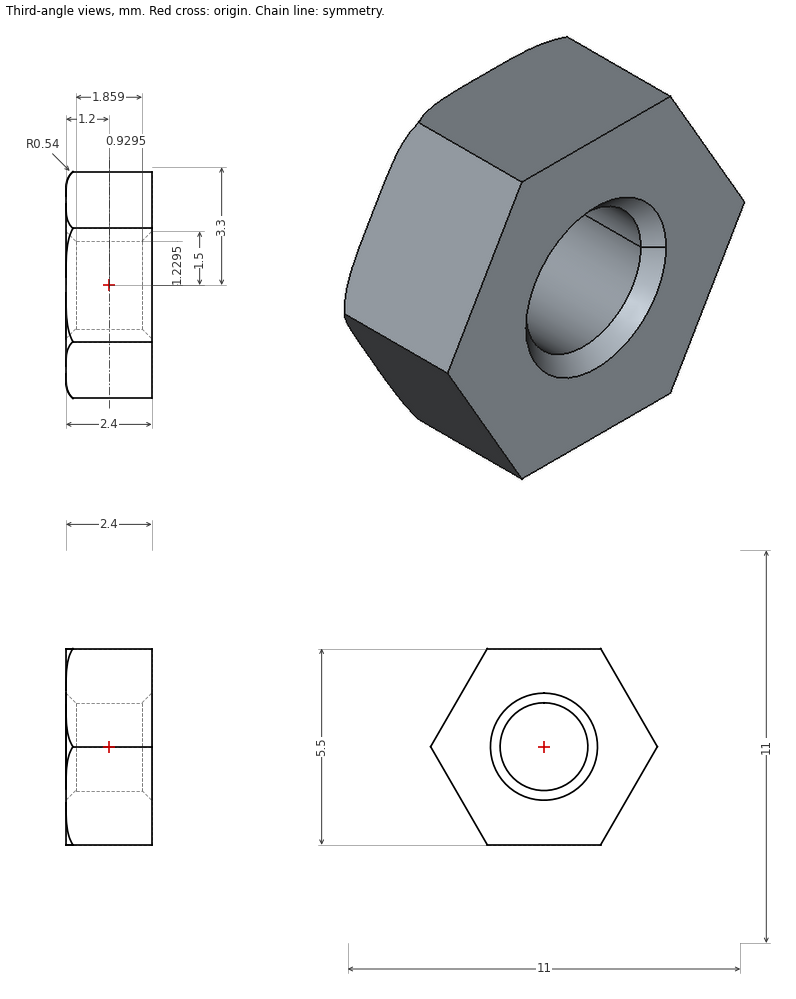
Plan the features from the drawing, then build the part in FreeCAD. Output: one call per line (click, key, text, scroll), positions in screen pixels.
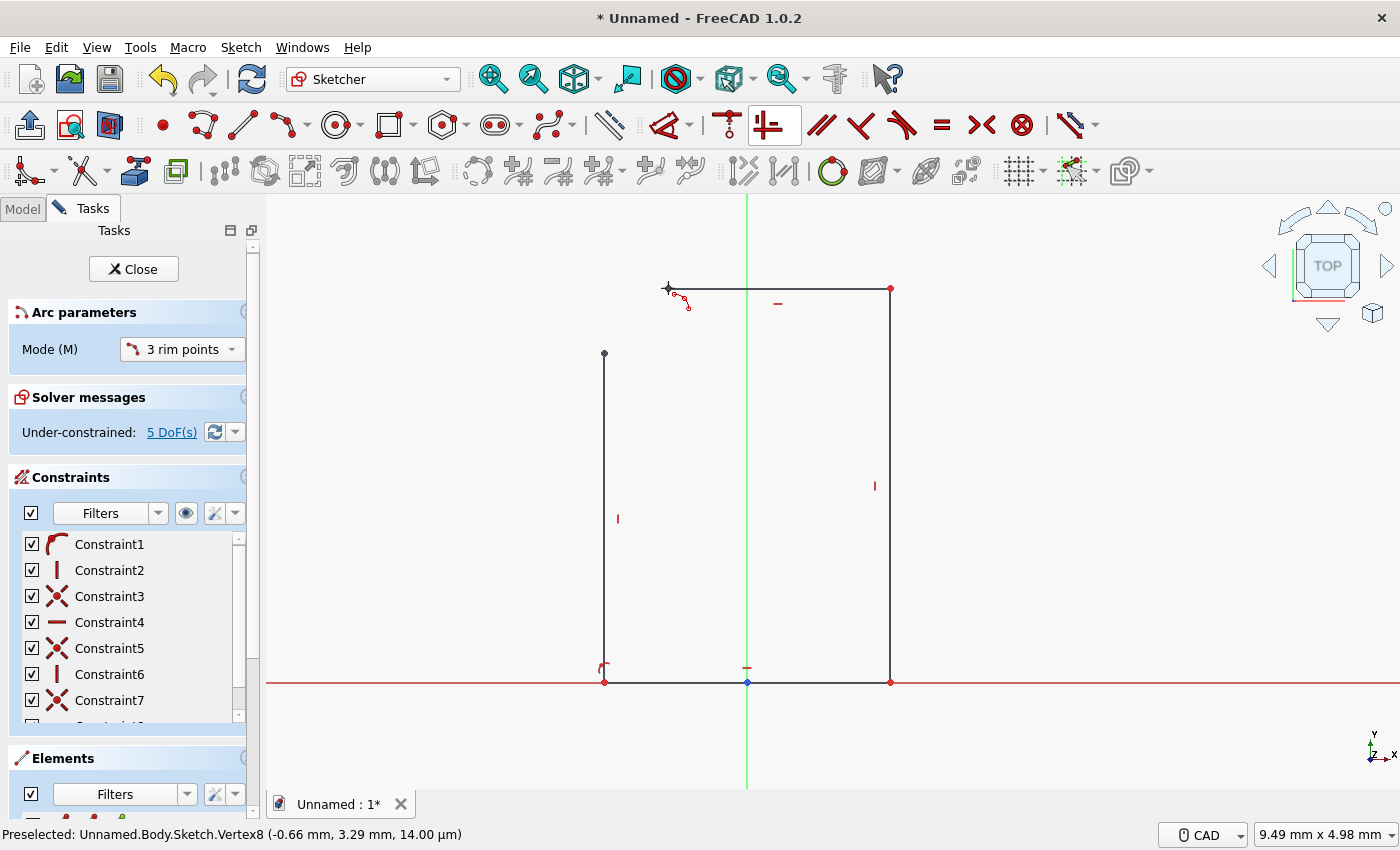
click(668, 289)
click(604, 354)
click(623, 307)
key(Escape)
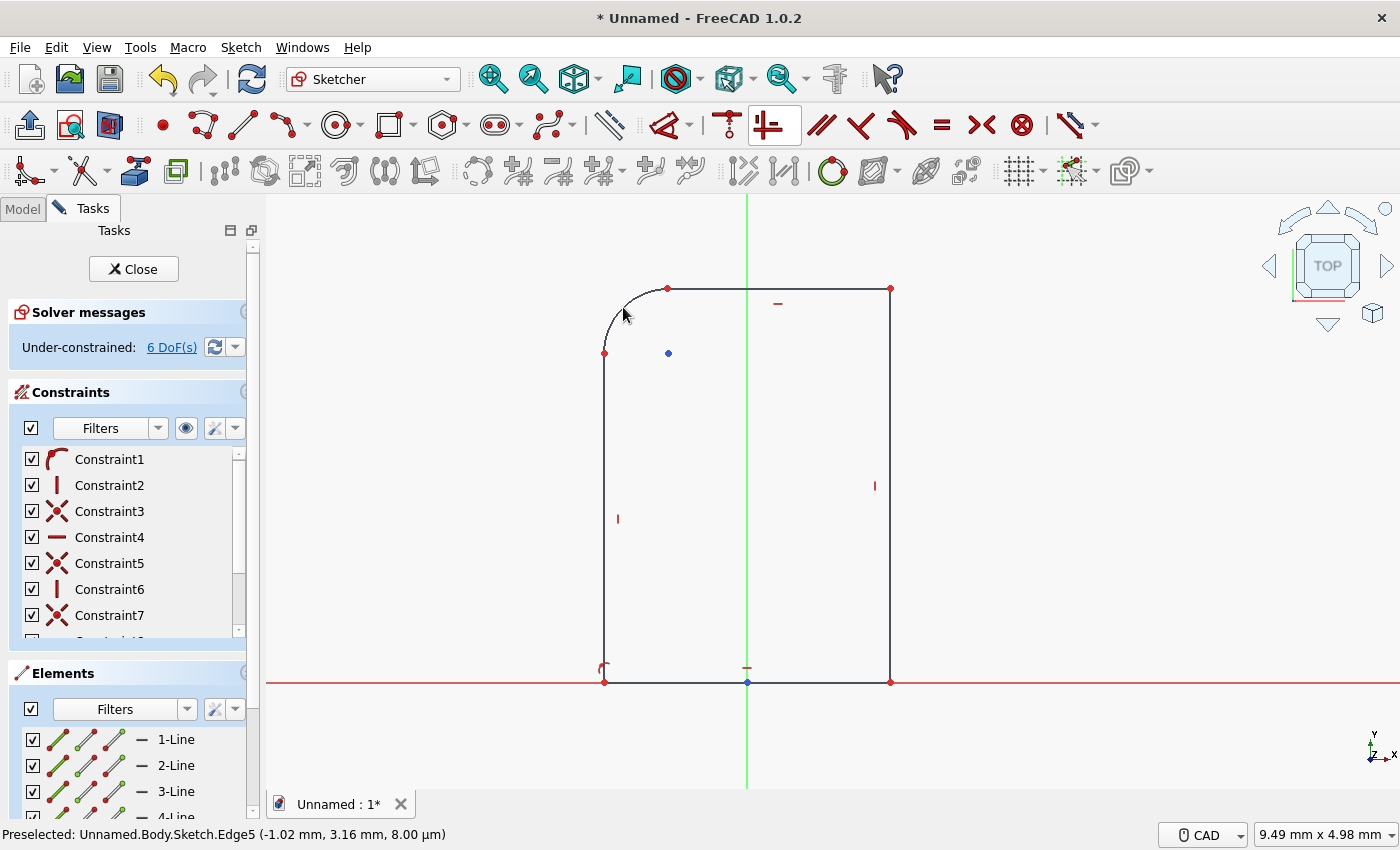
click(604, 453)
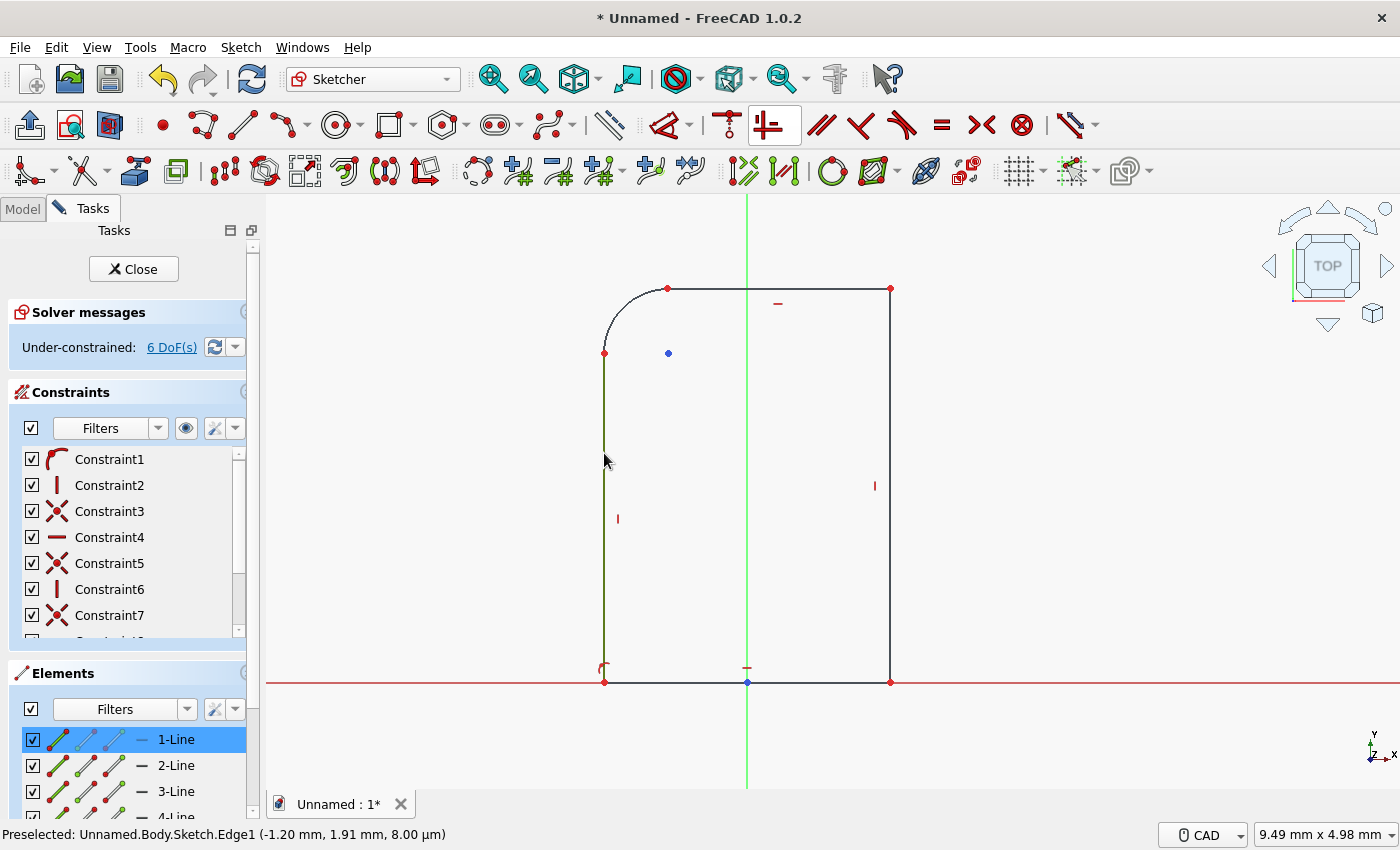
click(639, 296)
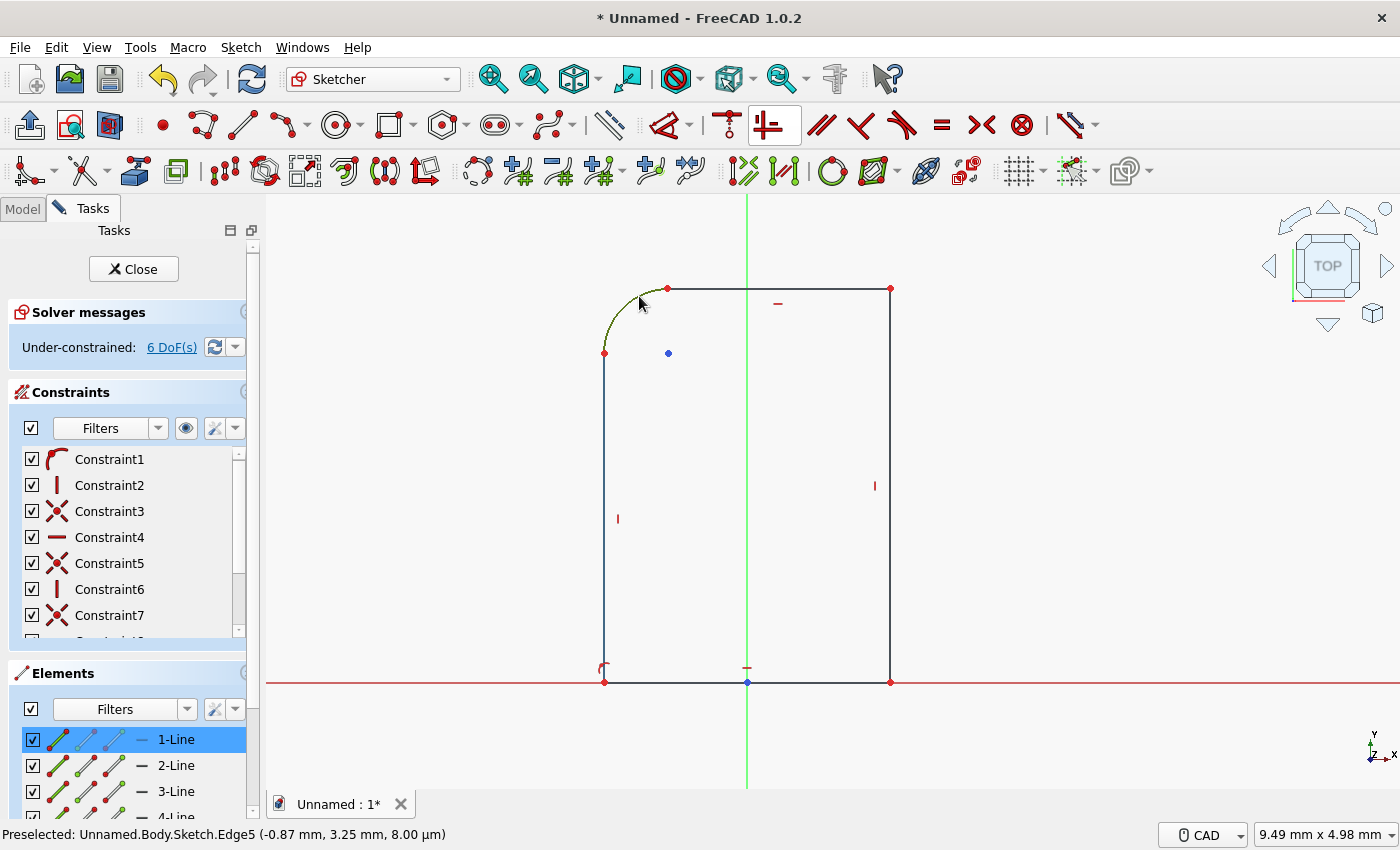
click(902, 126)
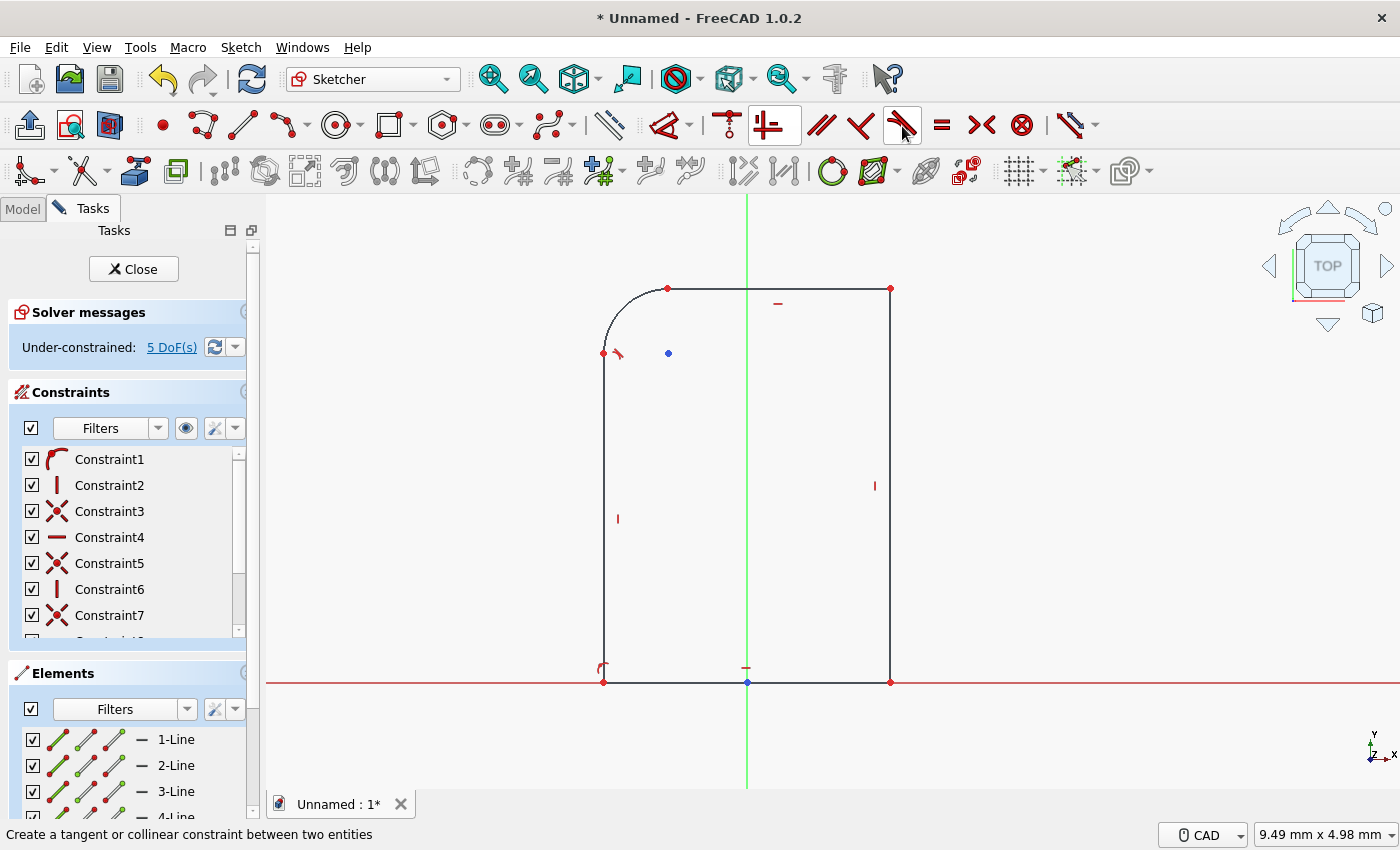
click(823, 289)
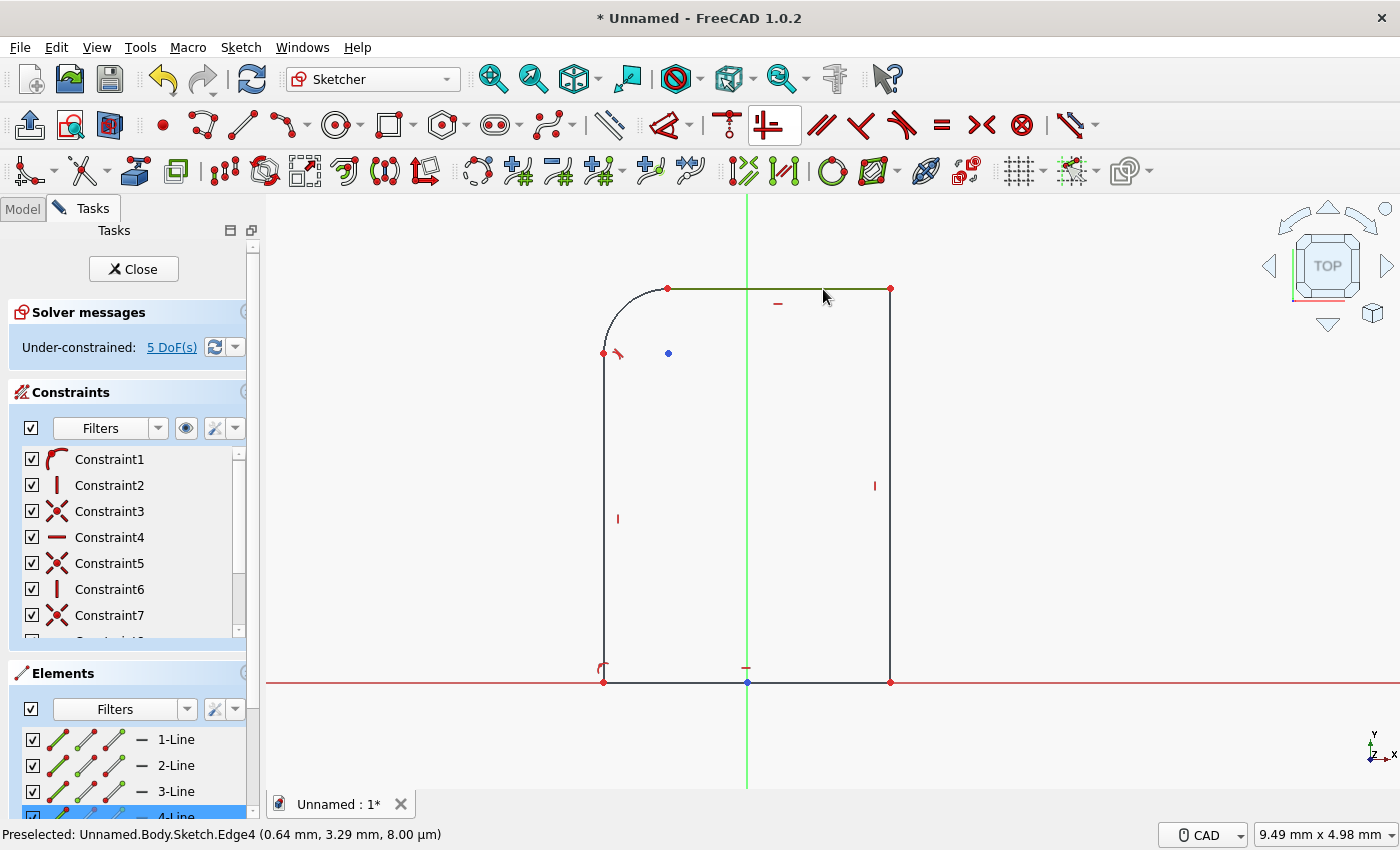
click(639, 296)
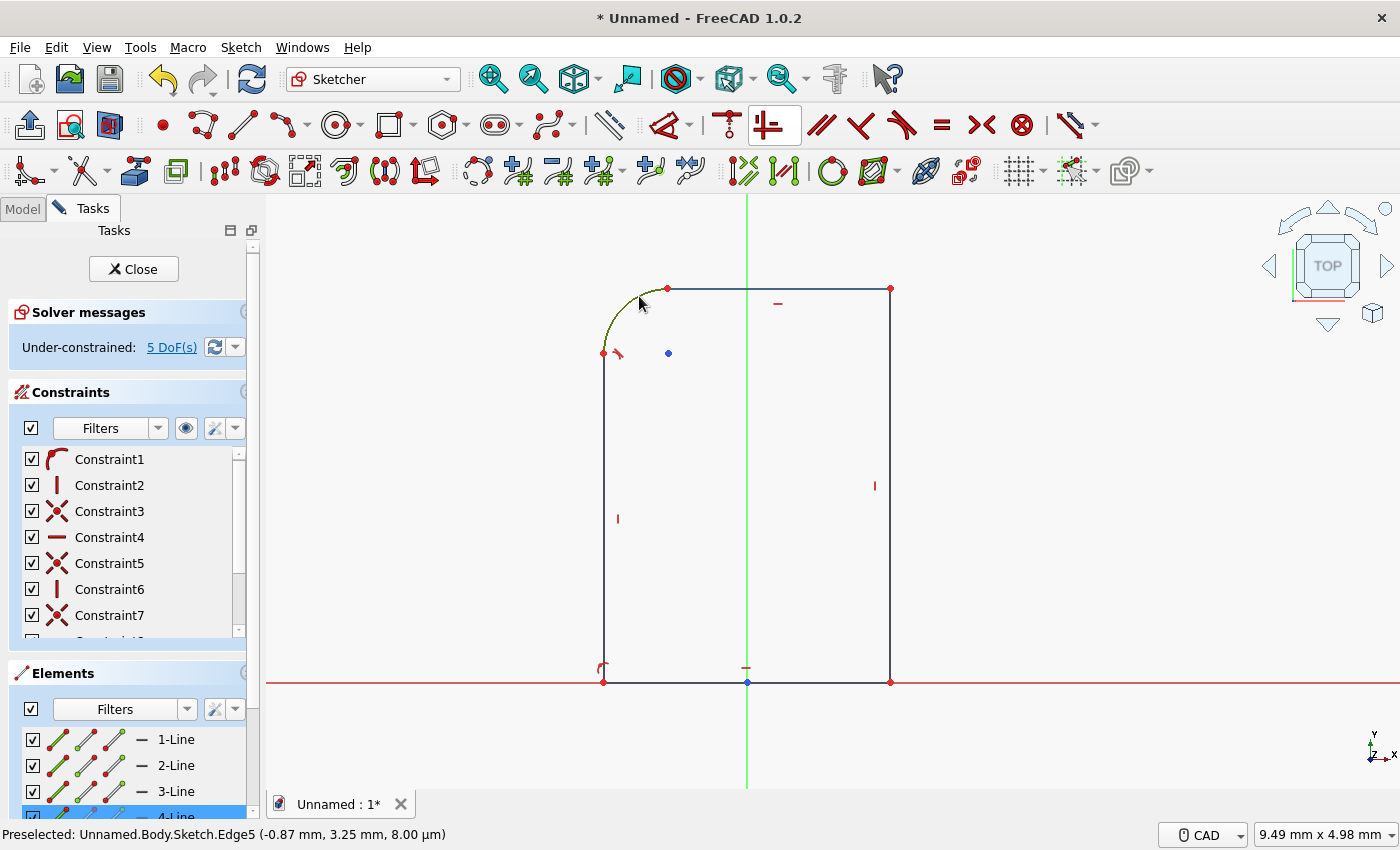
click(902, 126)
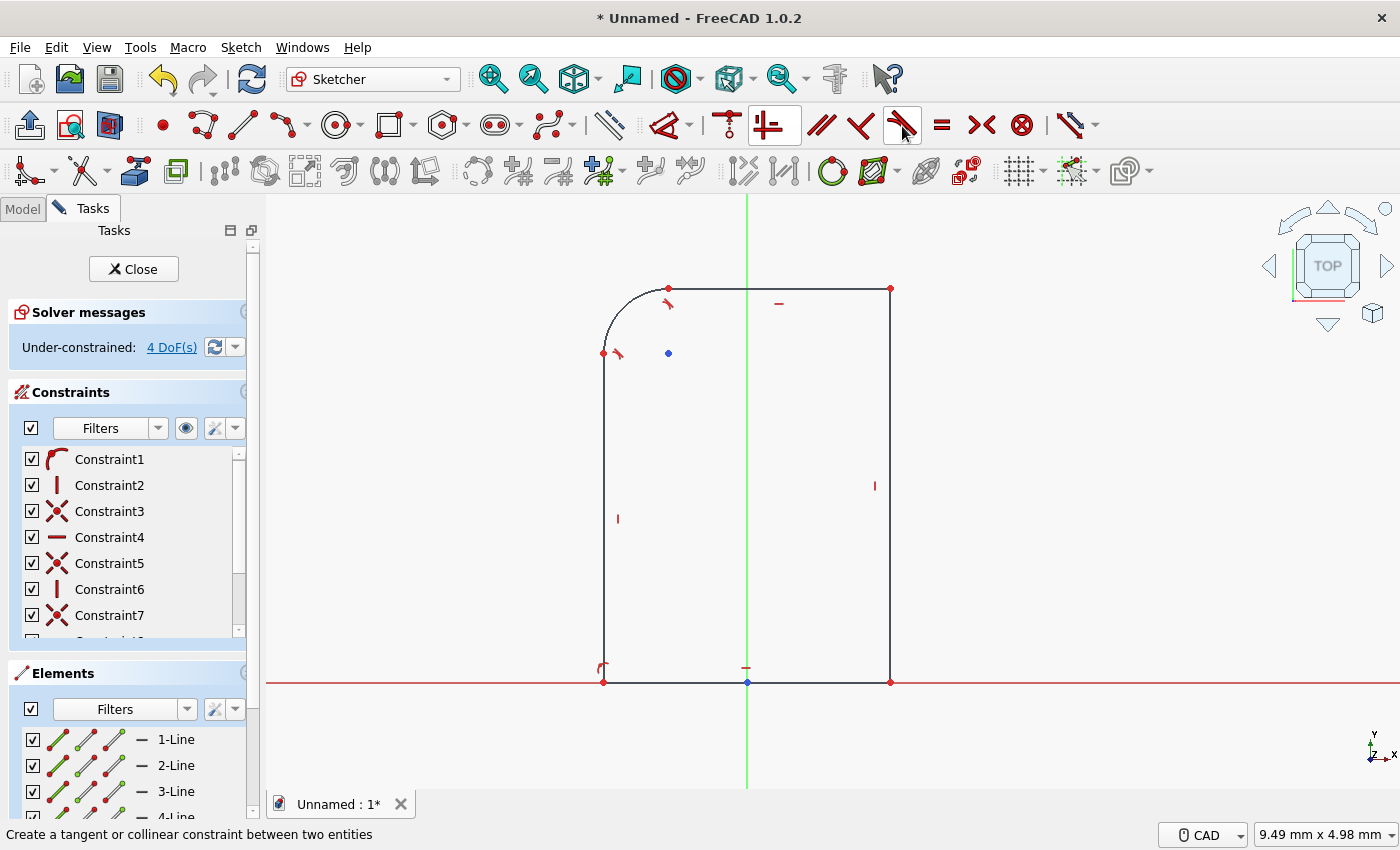
click(664, 126)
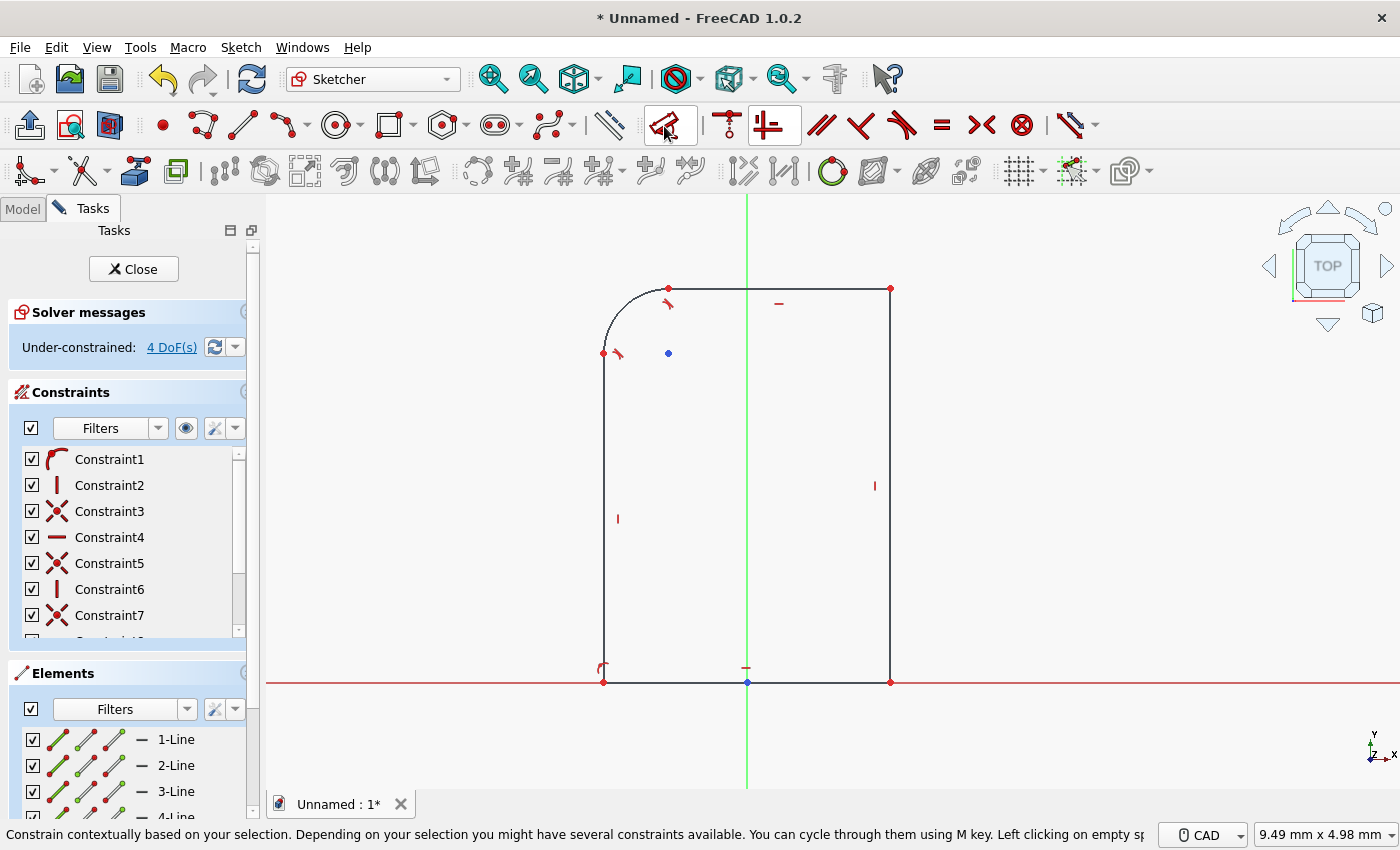
click(639, 296)
click(624, 268)